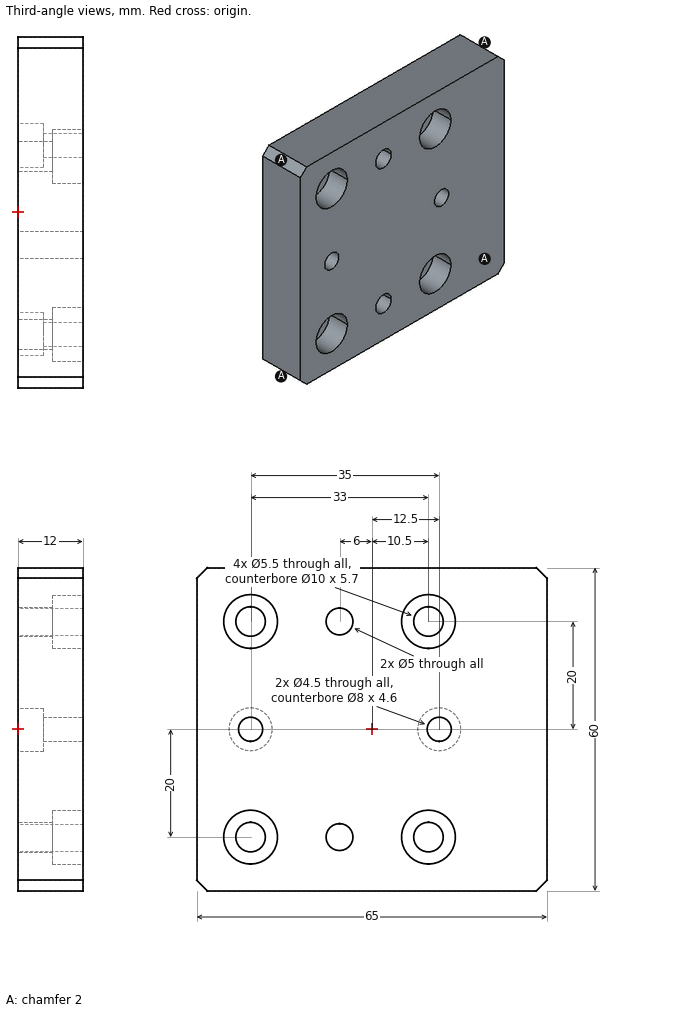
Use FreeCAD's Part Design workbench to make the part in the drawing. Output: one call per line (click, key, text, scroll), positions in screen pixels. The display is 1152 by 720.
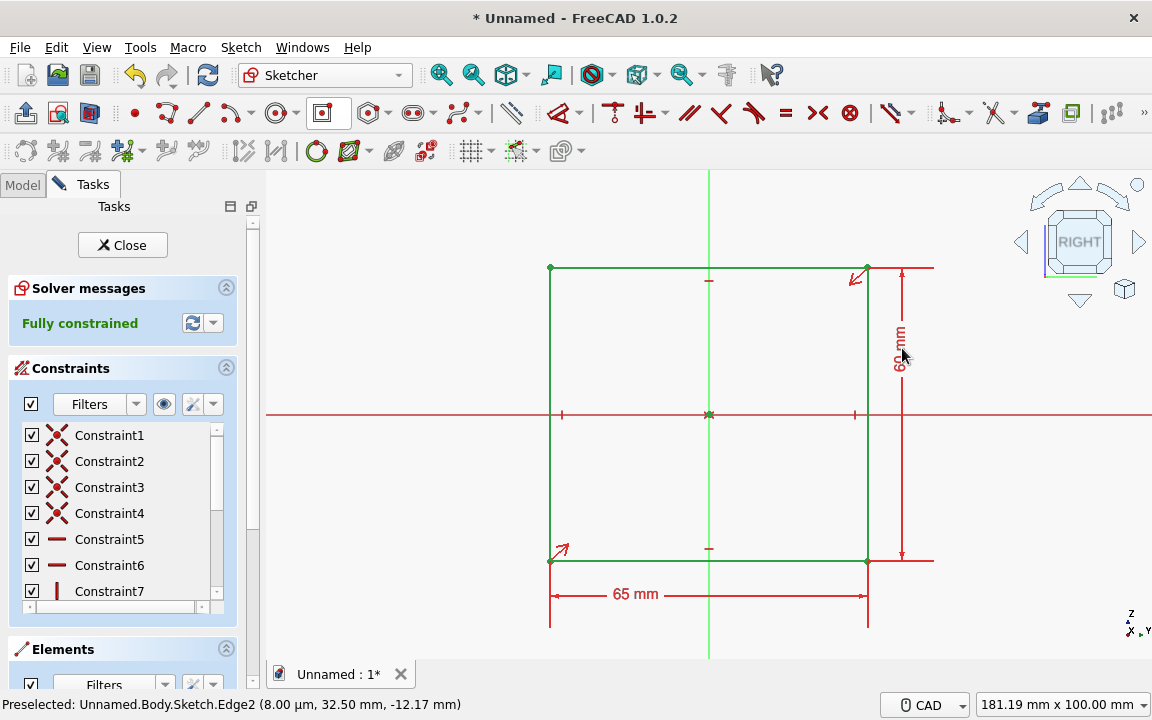
click(123, 245)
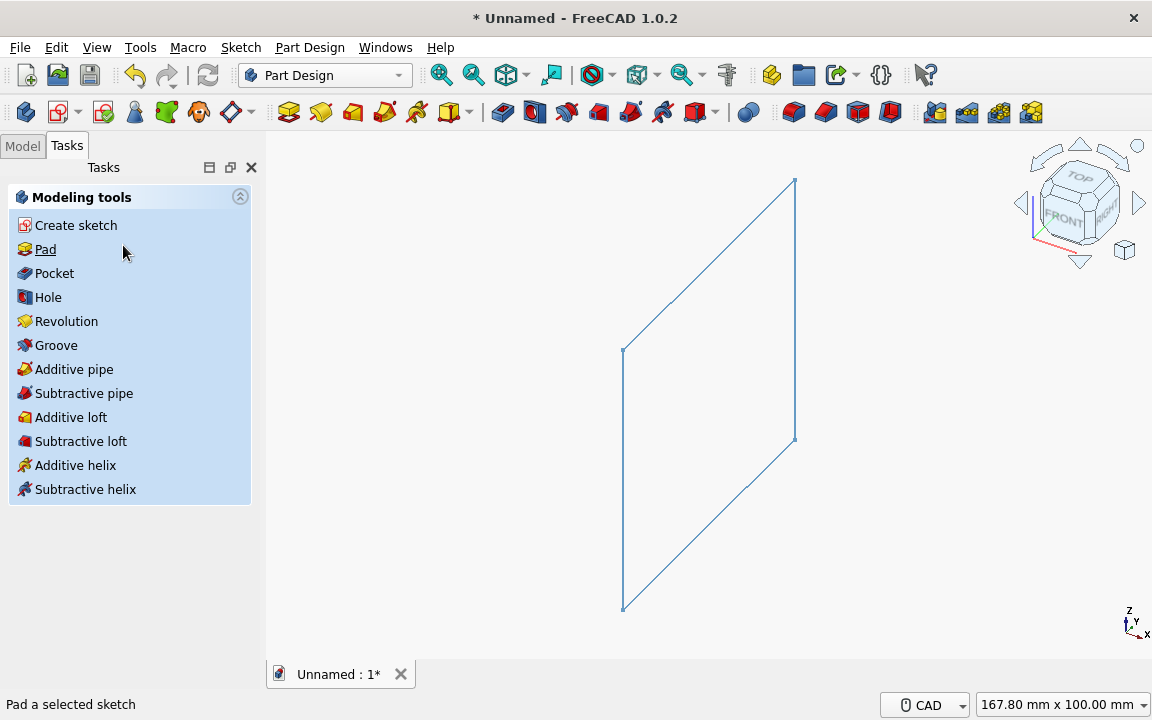
click(290, 112)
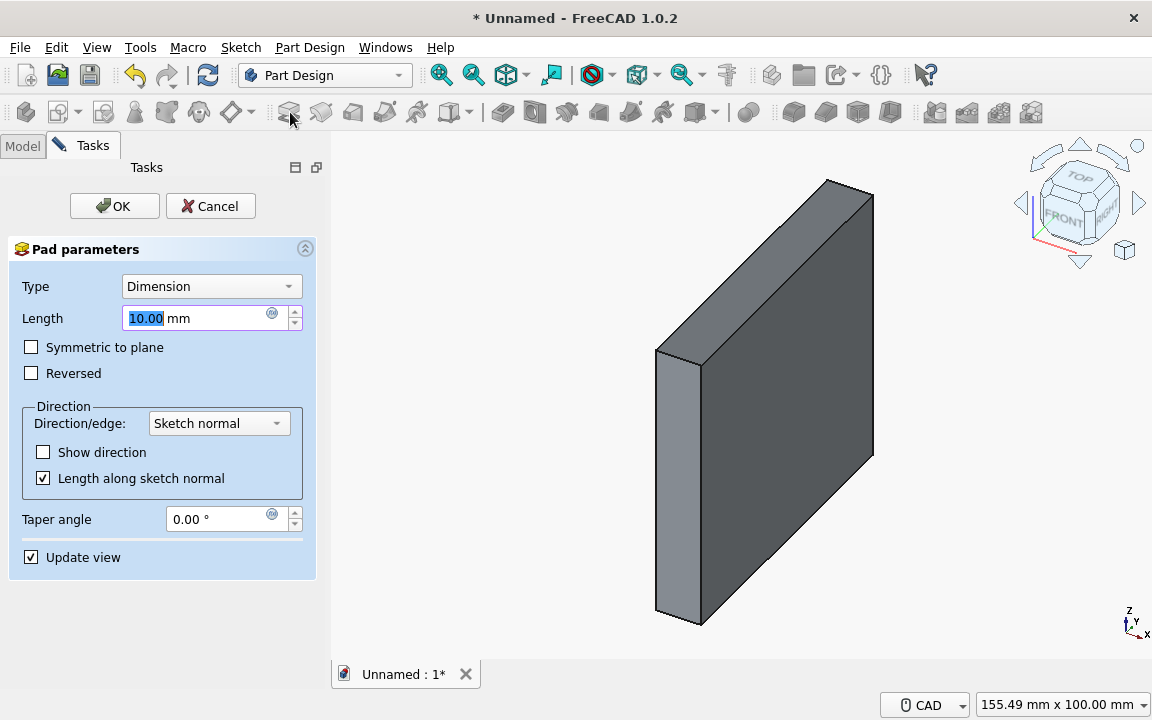
text(12)
key(Tab)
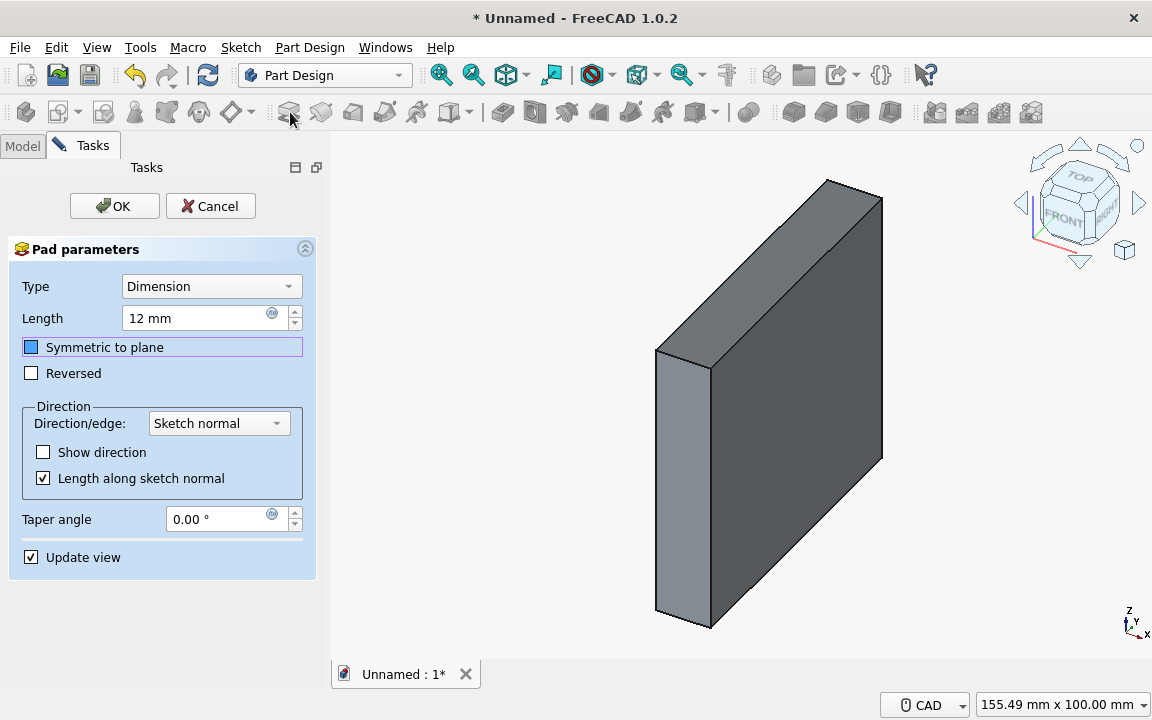
click(115, 206)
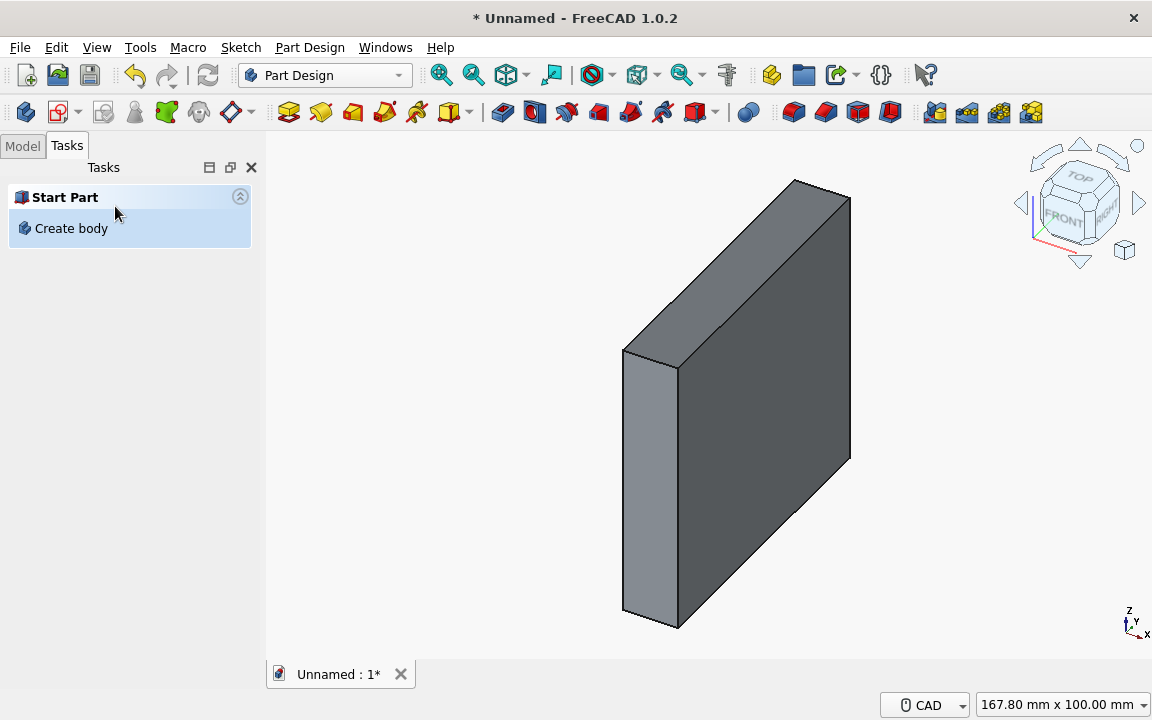
click(58, 112)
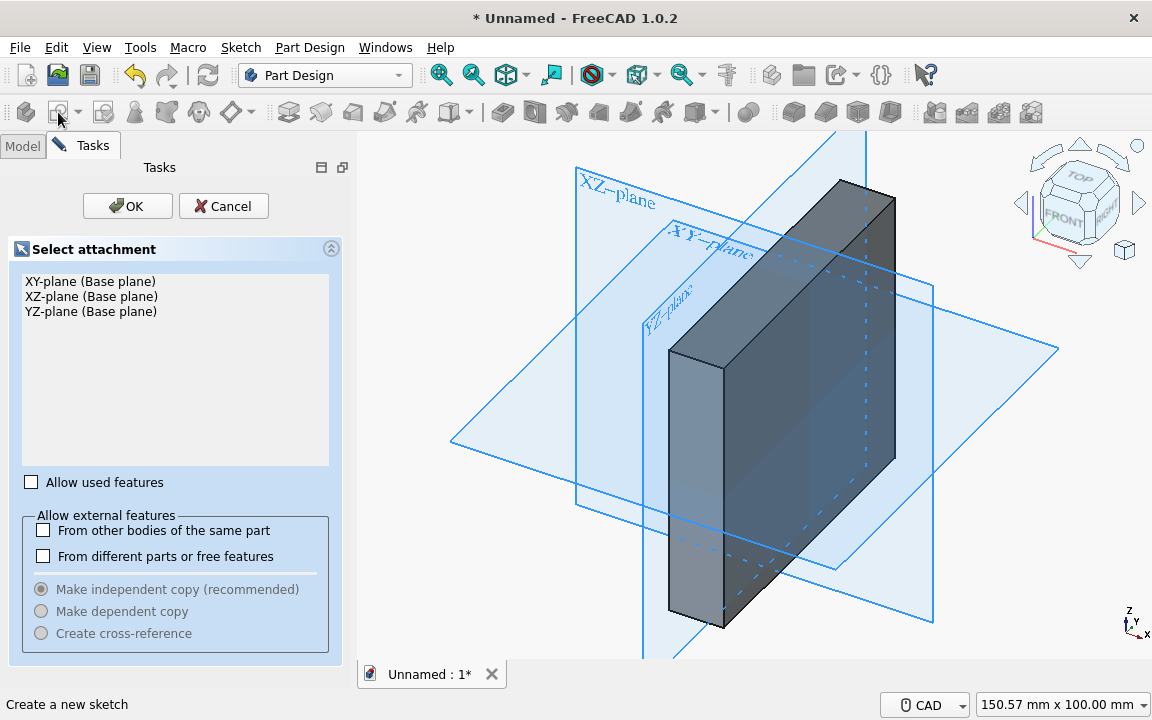
click(82, 312)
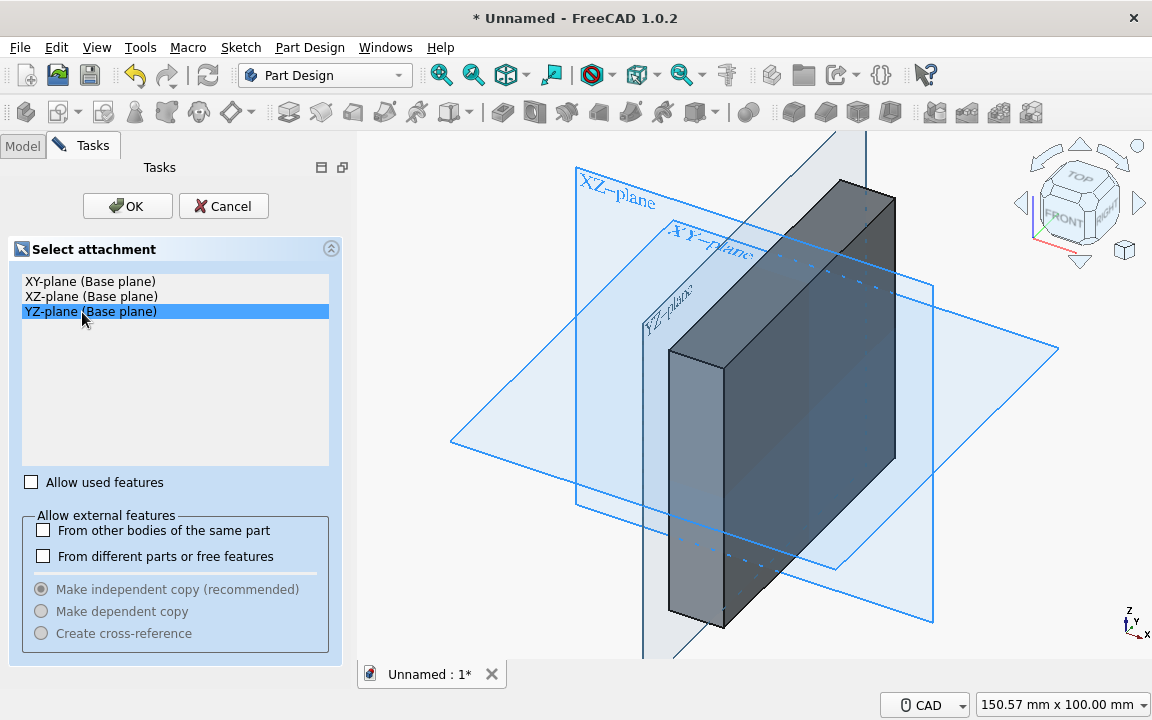
click(128, 206)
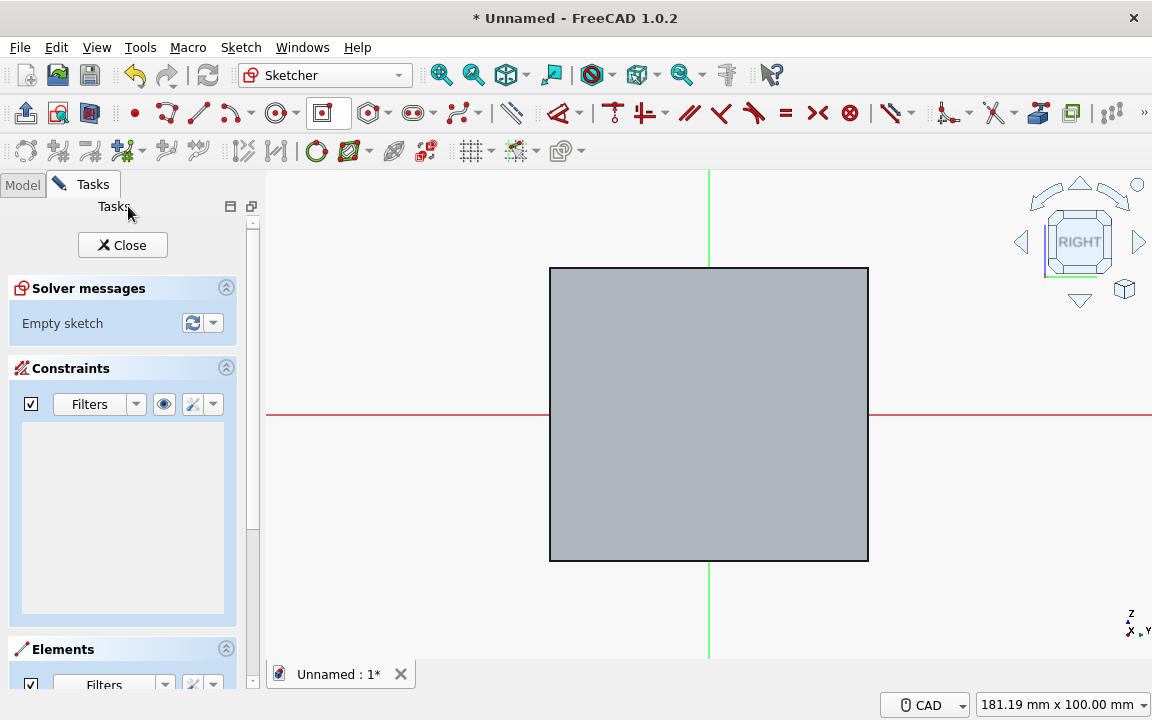
click(90, 114)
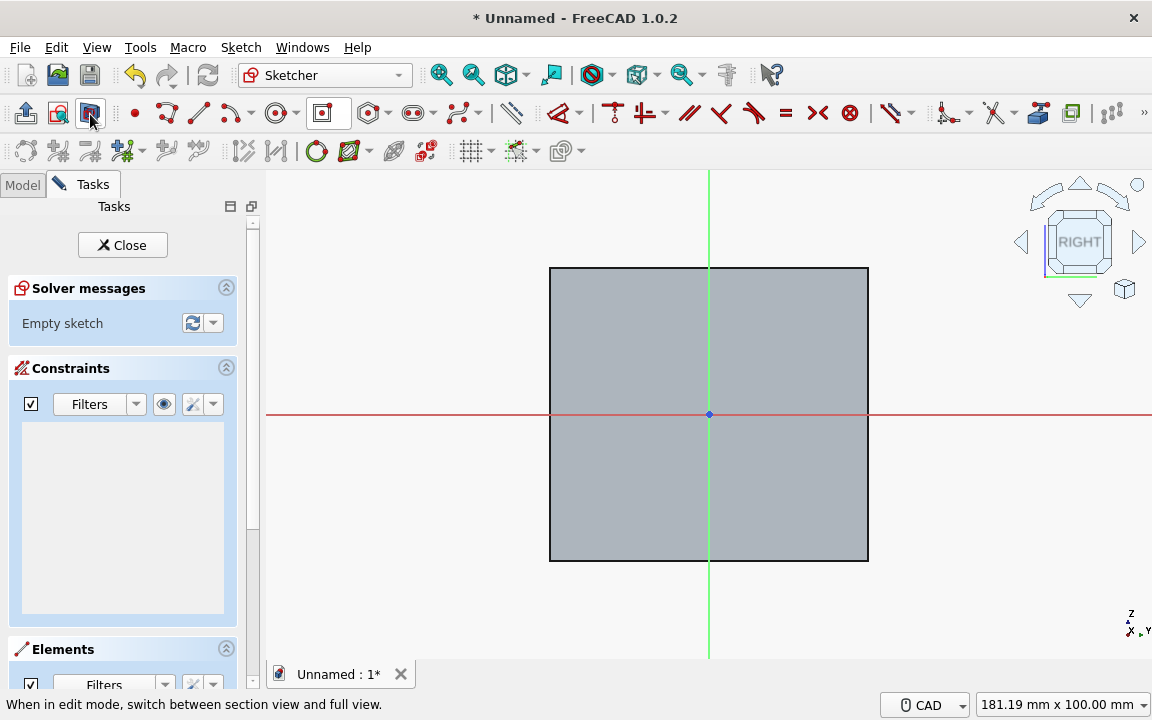
scroll(710, 415, up, 5)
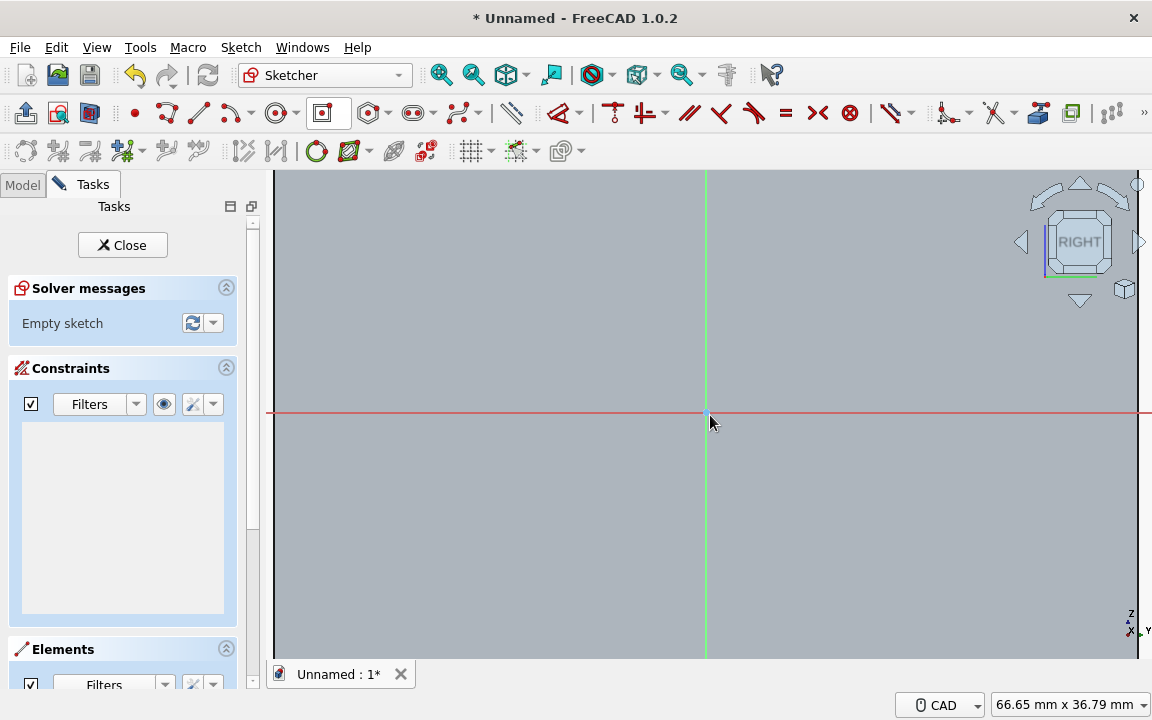
click(276, 114)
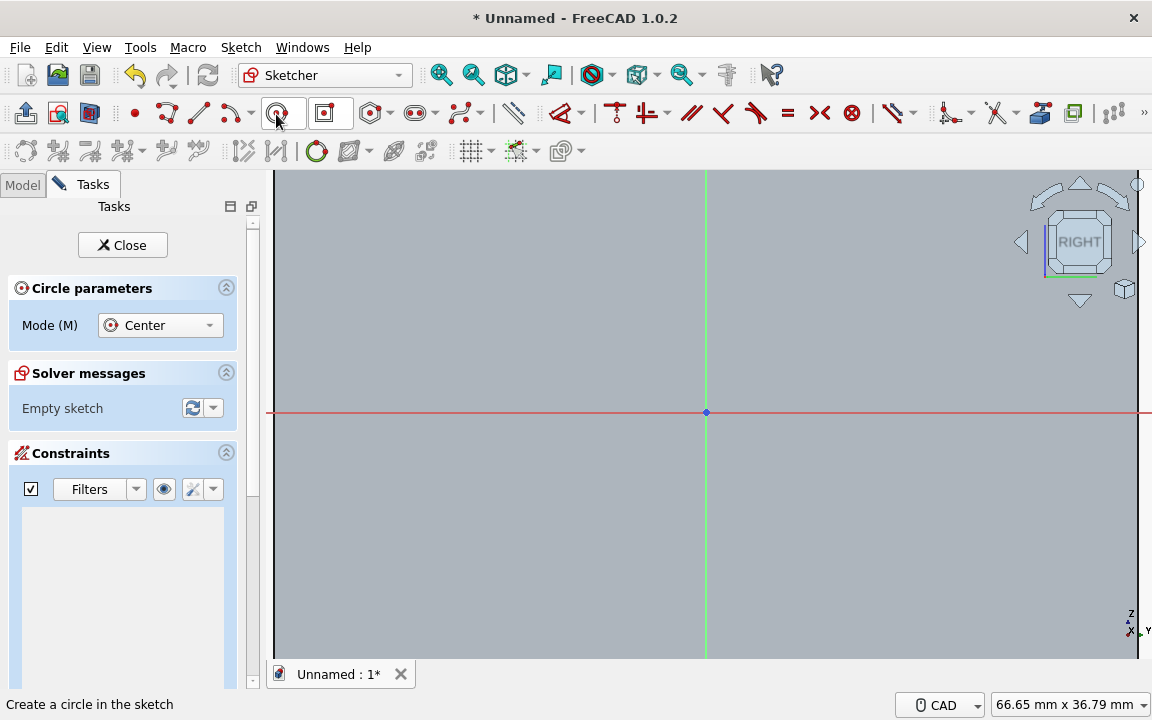
click(873, 413)
click(894, 392)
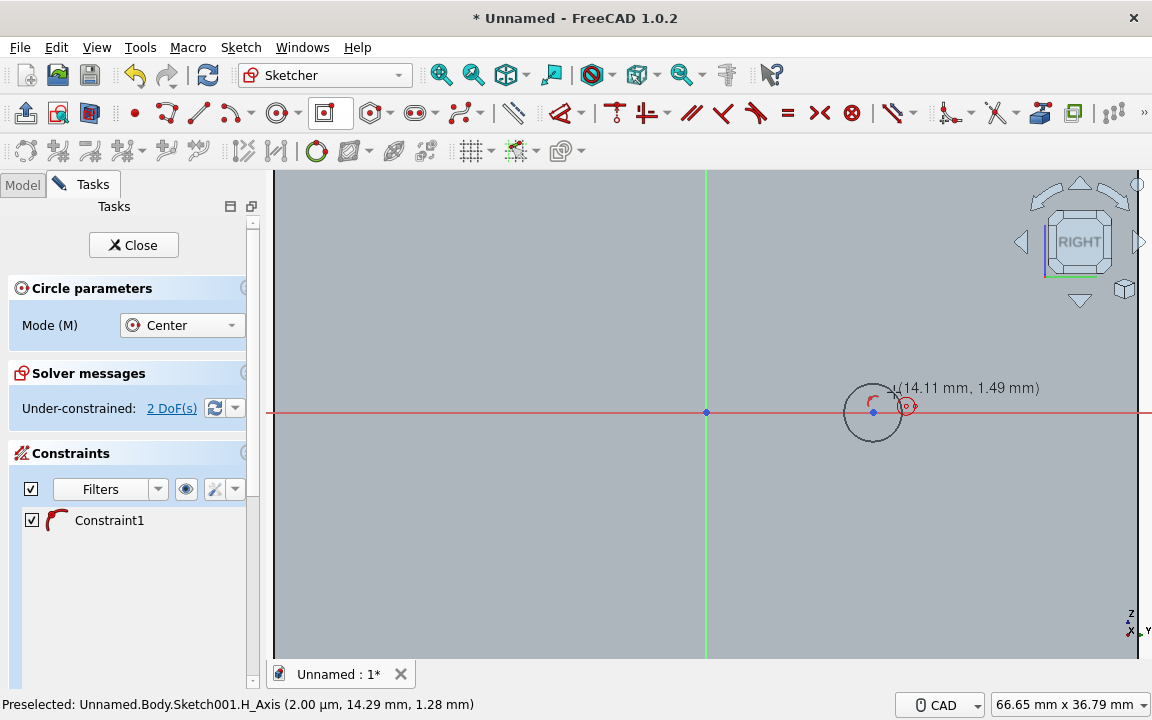
click(407, 413)
click(428, 392)
key(Escape)